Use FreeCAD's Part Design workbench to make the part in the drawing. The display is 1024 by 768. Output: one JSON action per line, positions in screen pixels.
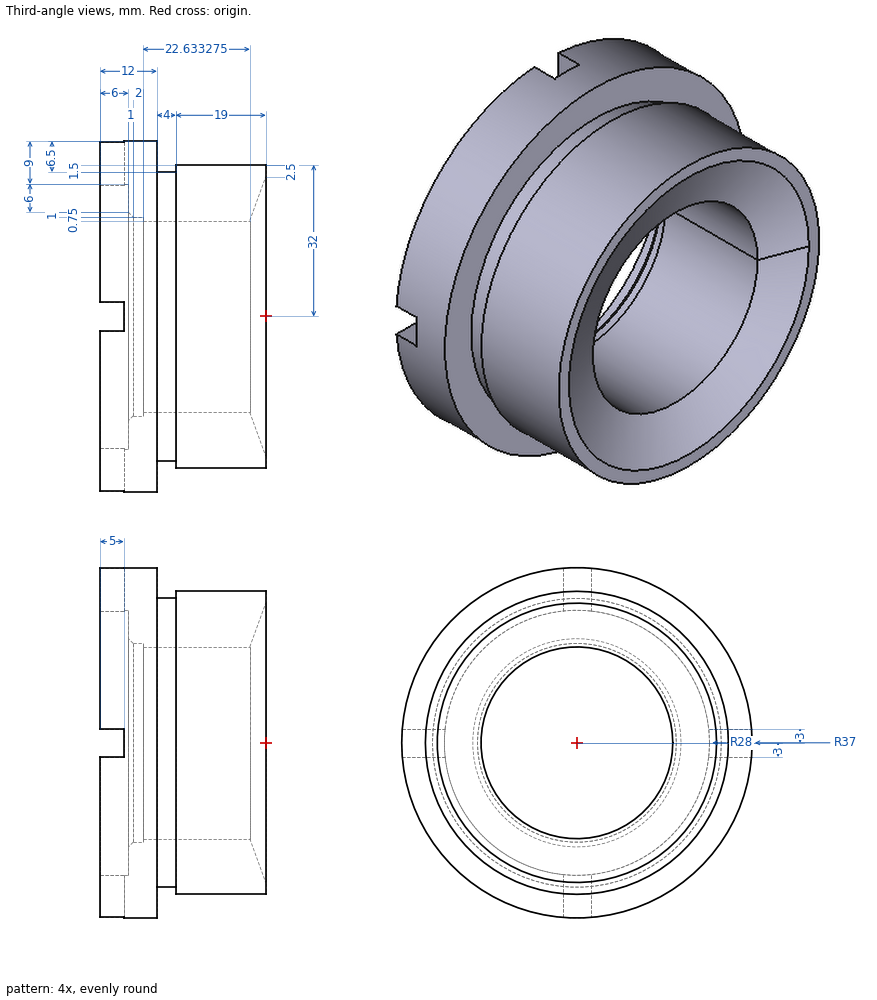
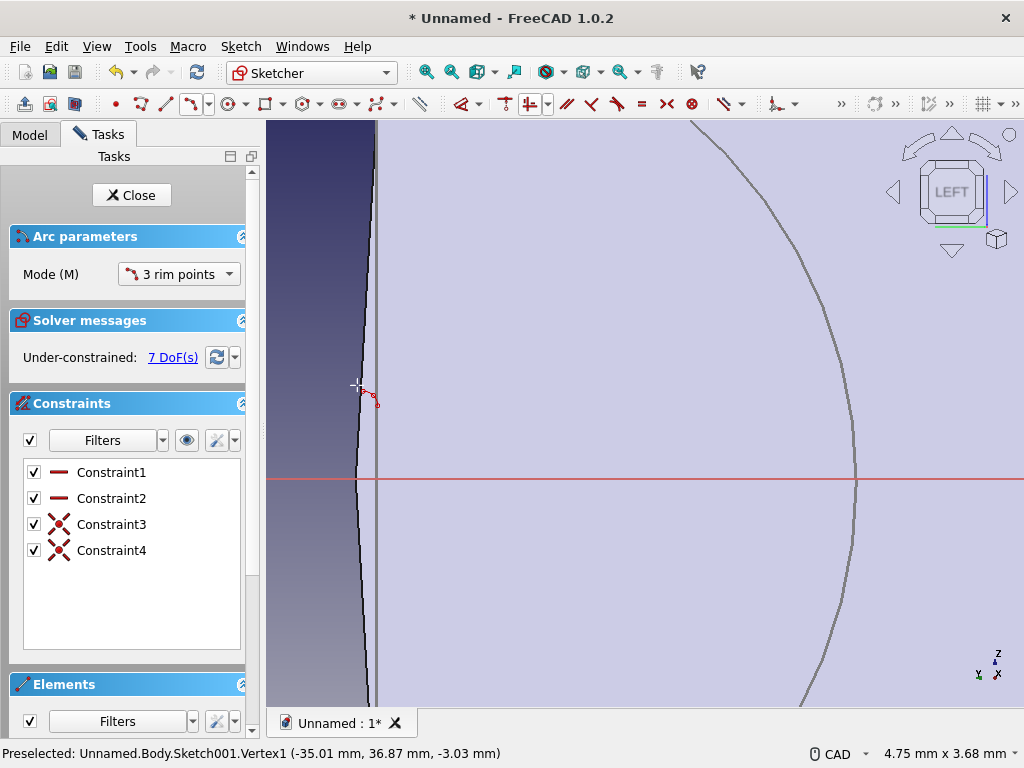
{"action": "left_click", "coordinate": [357, 384]}
{"action": "key", "text": "Escape"}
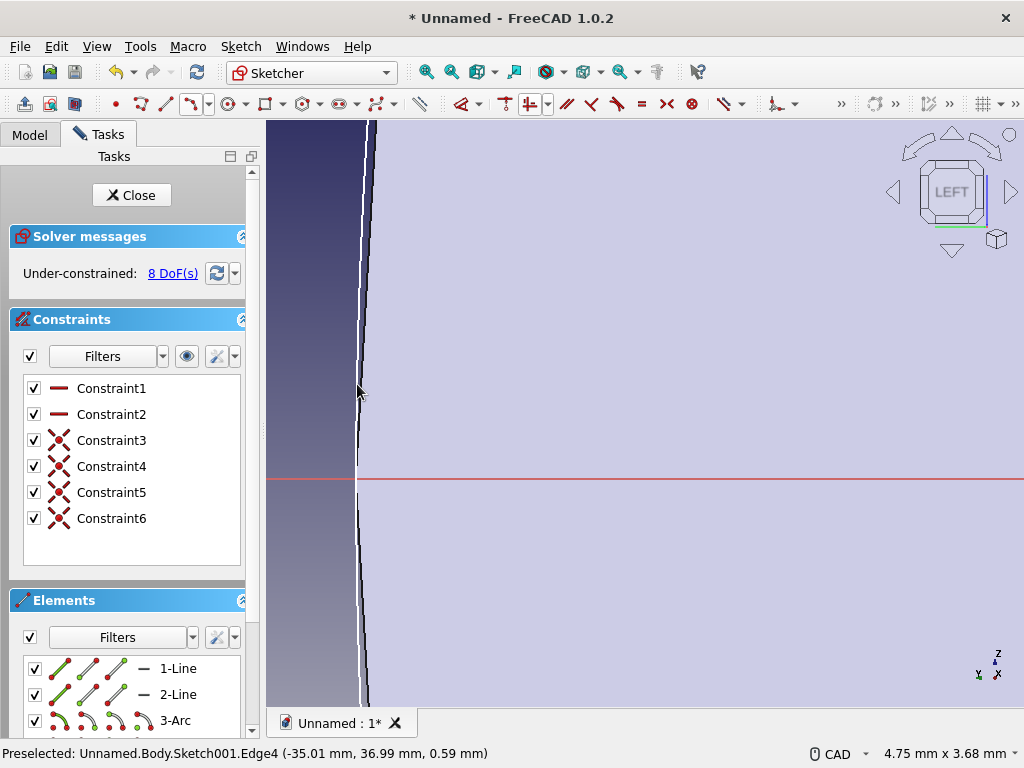
{"action": "scroll", "coordinate": [357, 385], "scroll_direction": "down", "scroll_amount": 6}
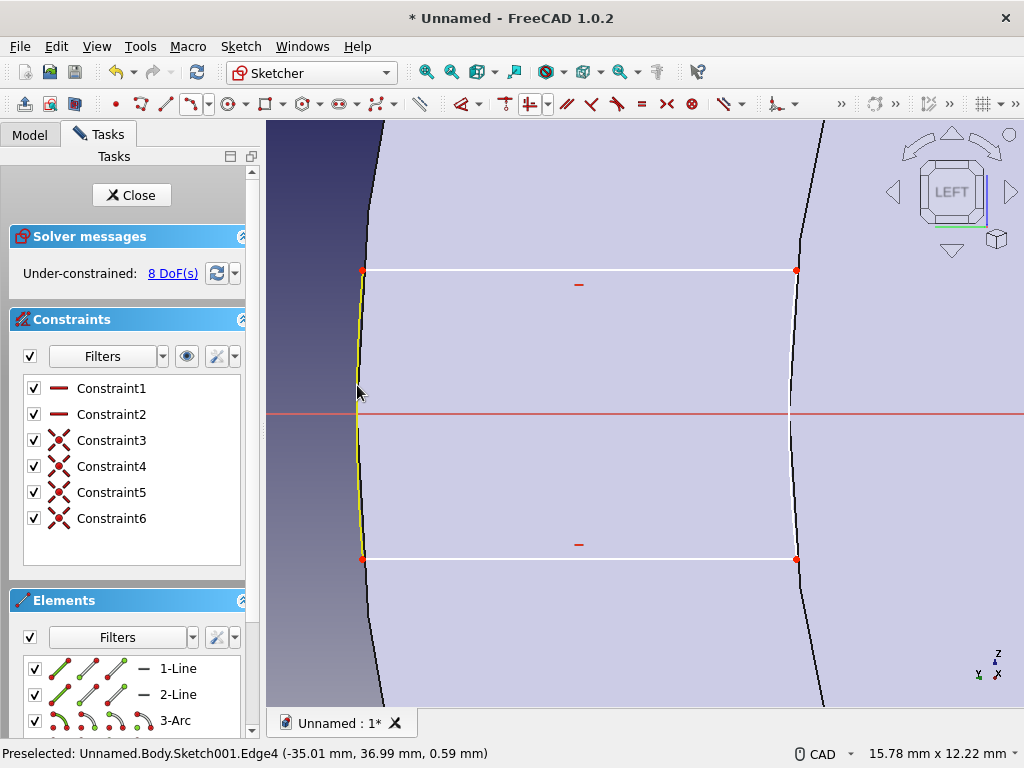
{"action": "left_click", "coordinate": [790, 357]}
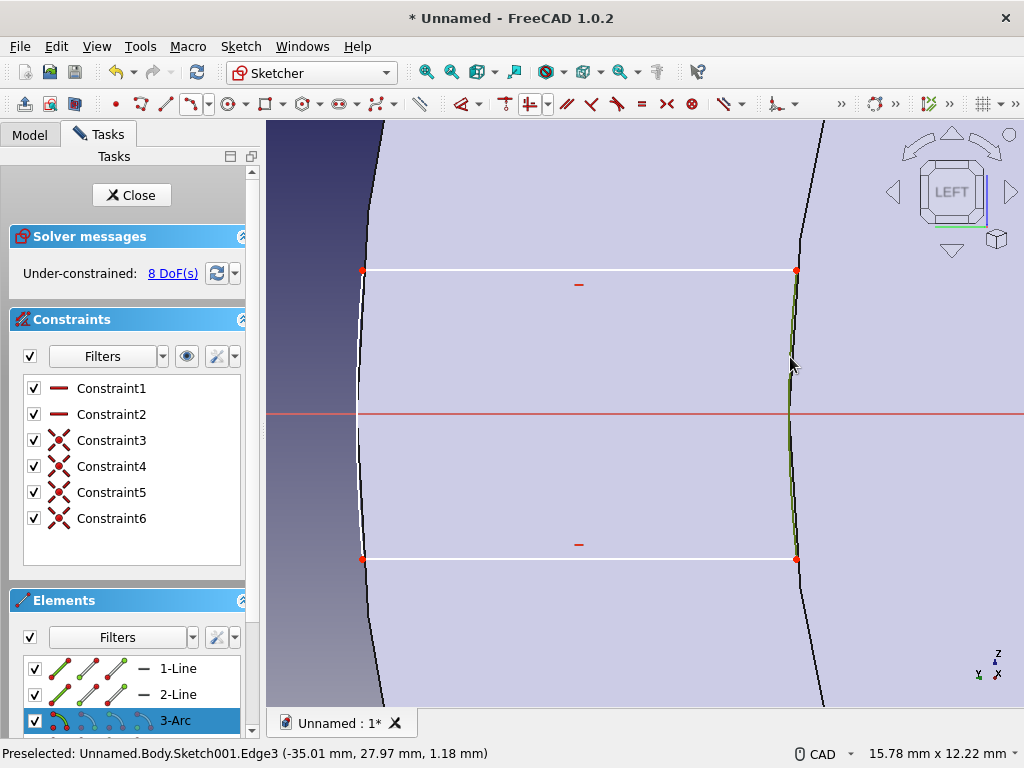
{"action": "left_click", "coordinate": [358, 357]}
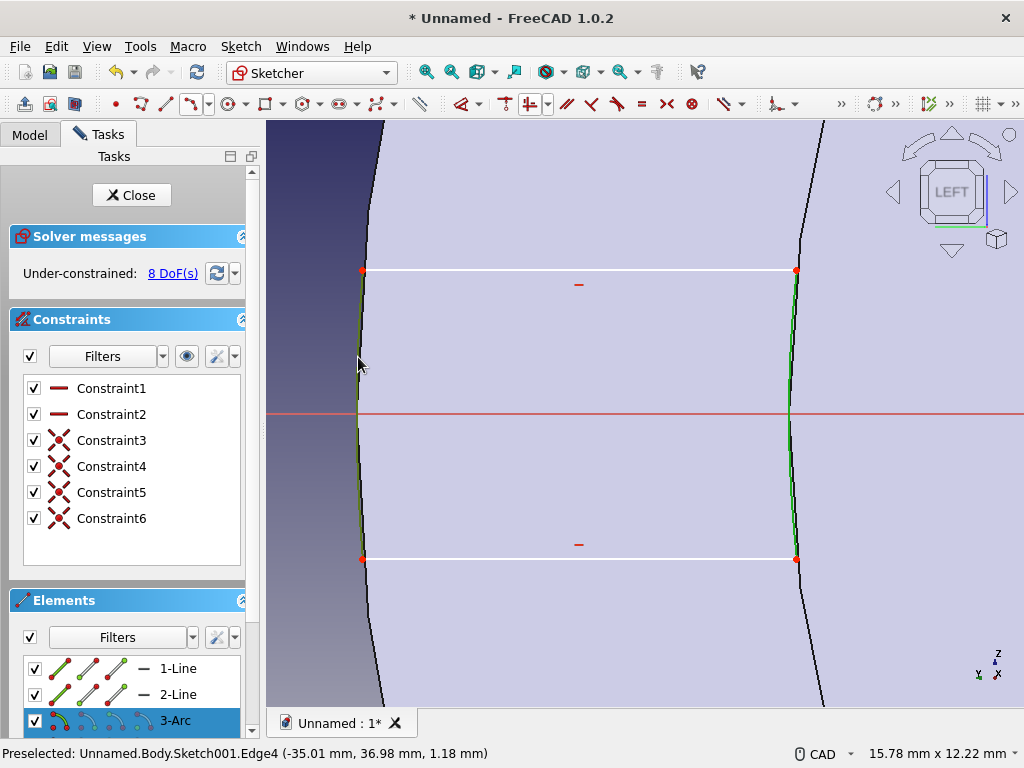
{"action": "left_click", "coordinate": [505, 104]}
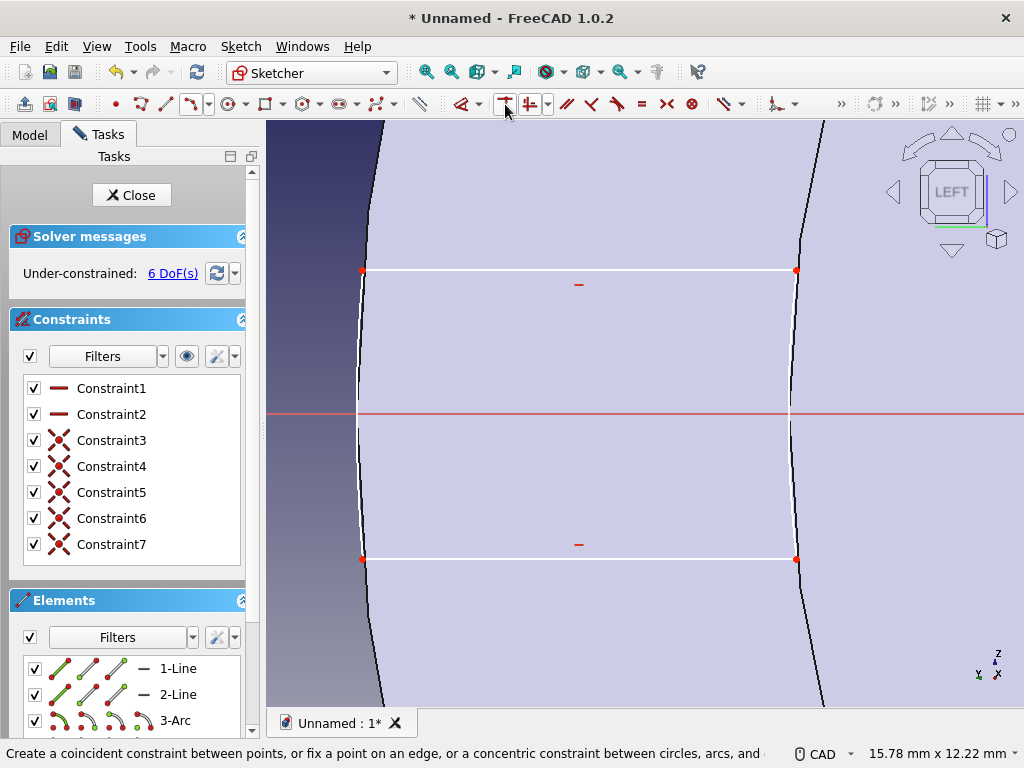
{"action": "scroll", "coordinate": [363, 413], "scroll_direction": "down", "scroll_amount": 7}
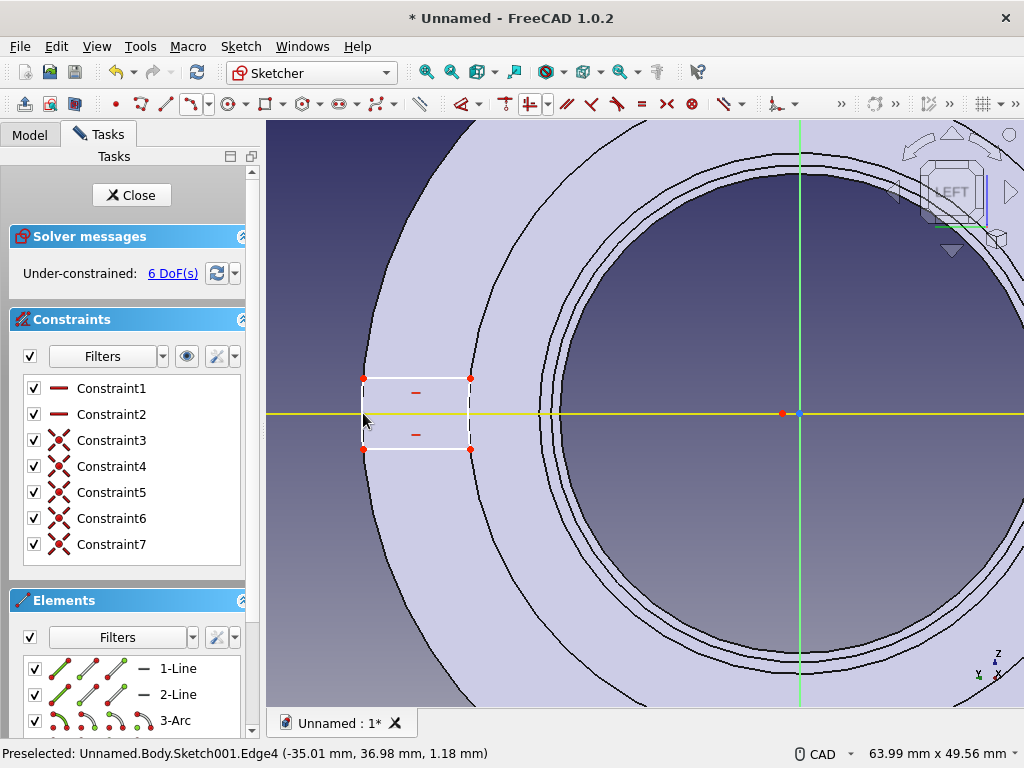
{"action": "left_click_drag", "start_coordinate": [772, 404], "coordinate": [810, 424]}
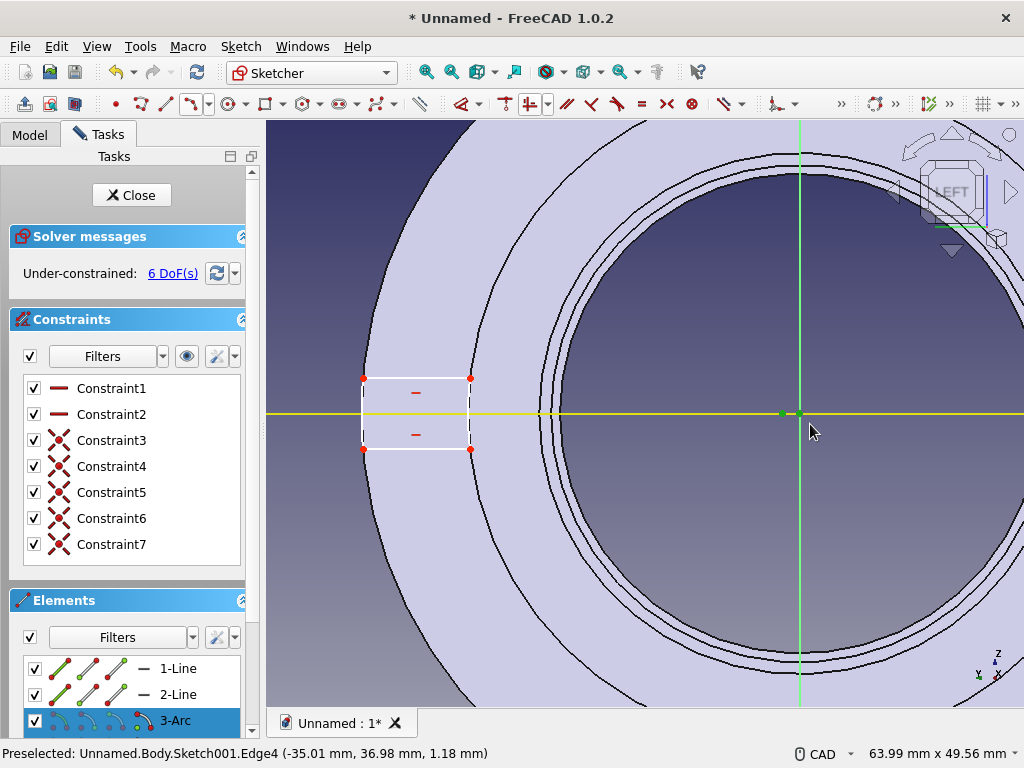
{"action": "left_click", "coordinate": [505, 104]}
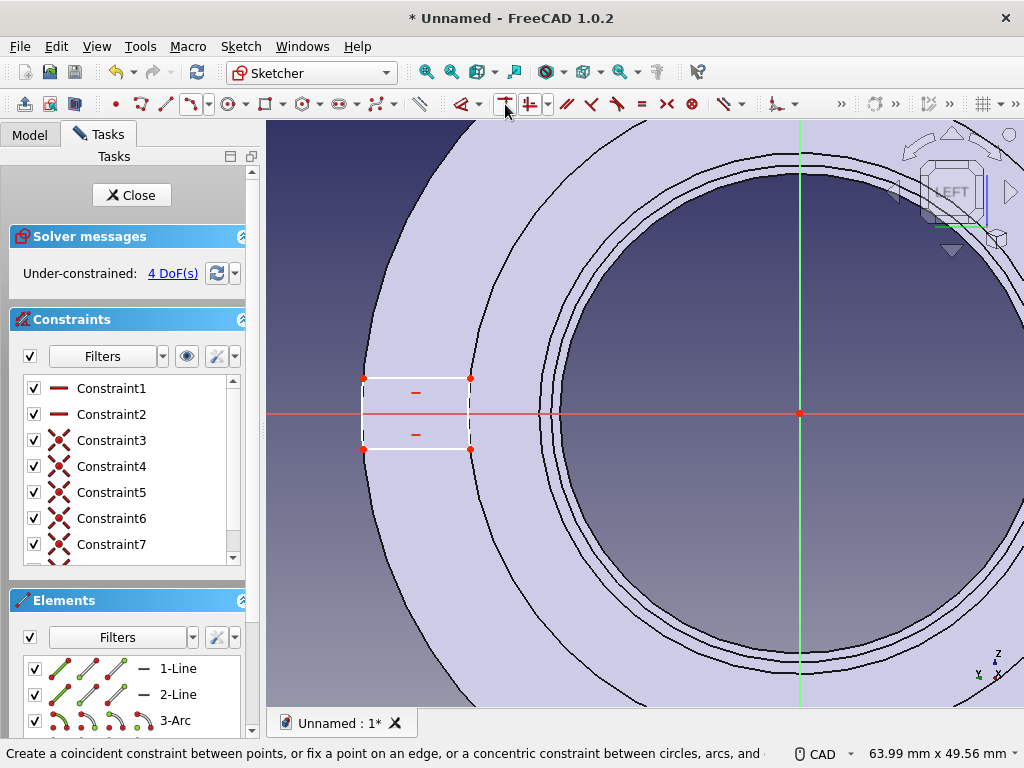
{"action": "left_click", "coordinate": [460, 104]}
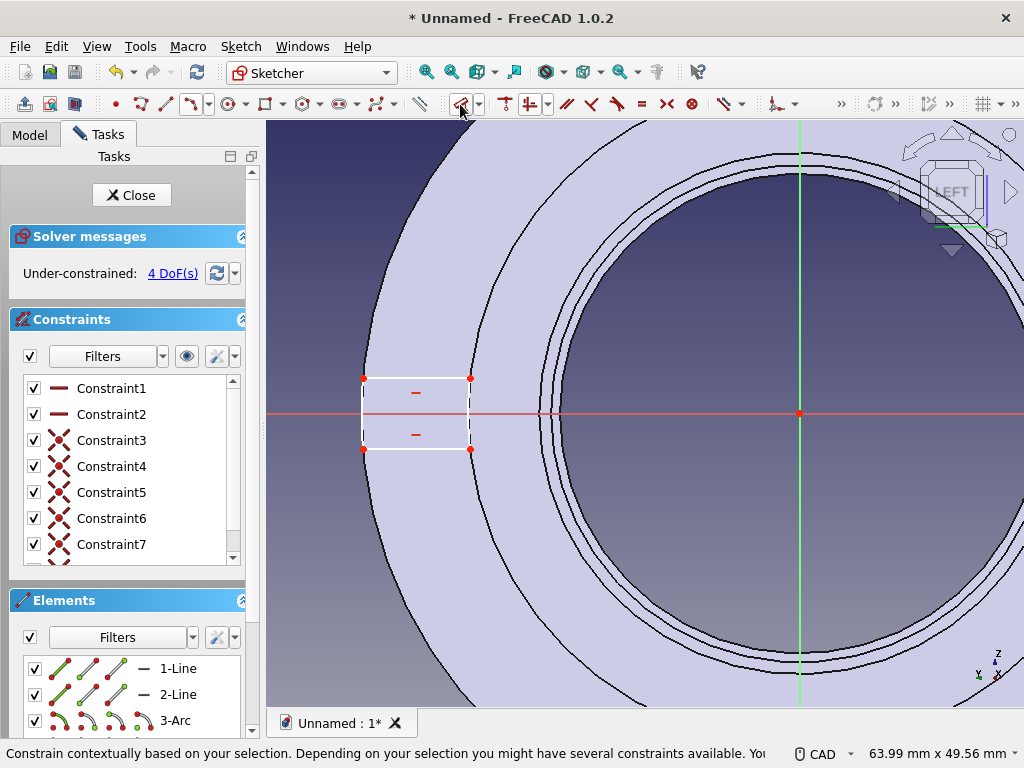
{"action": "left_click", "coordinate": [468, 400]}
{"action": "left_click", "coordinate": [436, 399]}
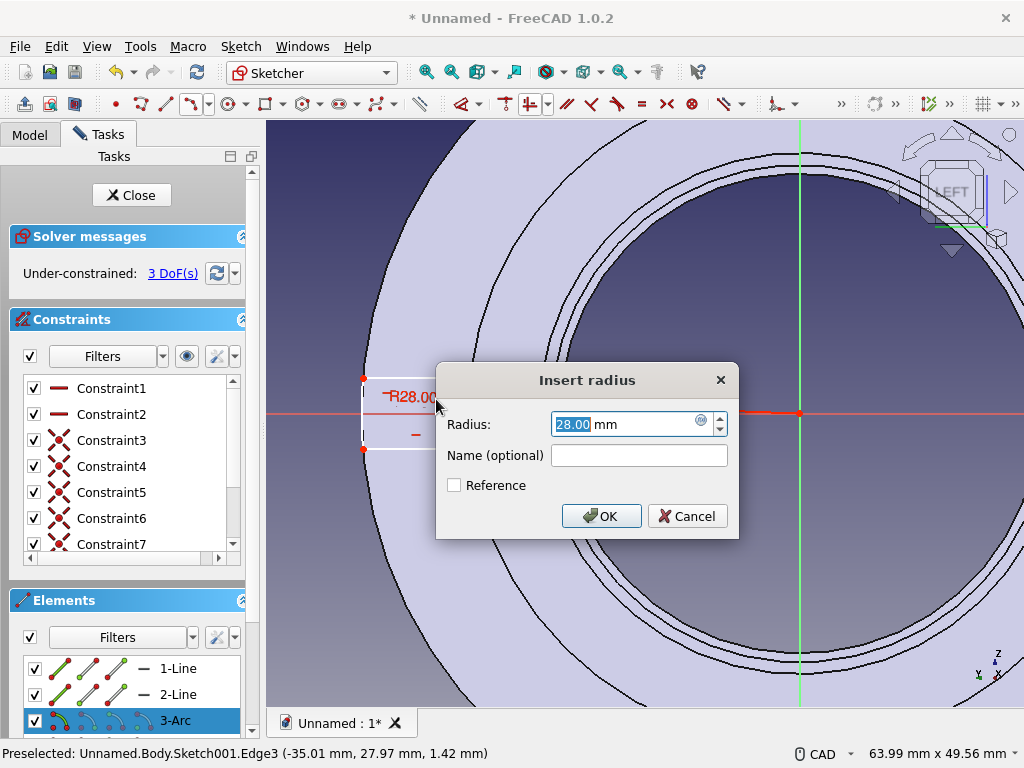
{"action": "type", "text": "28"}
{"action": "key", "text": "Return"}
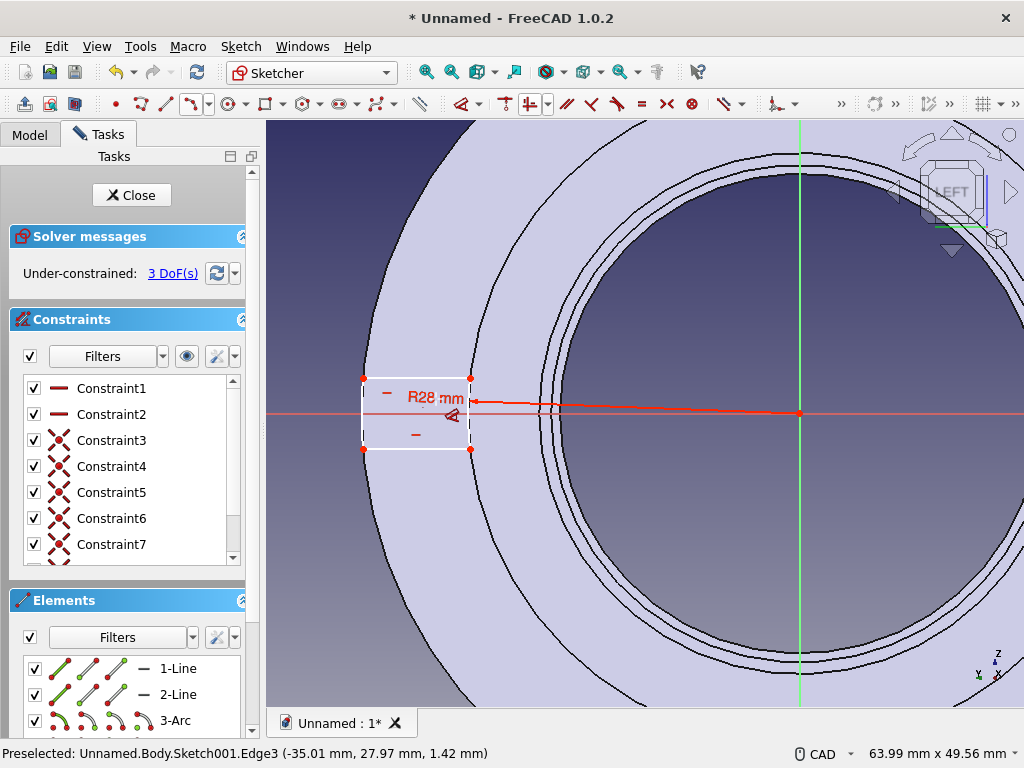
{"action": "left_click", "coordinate": [362, 400]}
{"action": "left_click", "coordinate": [330, 399]}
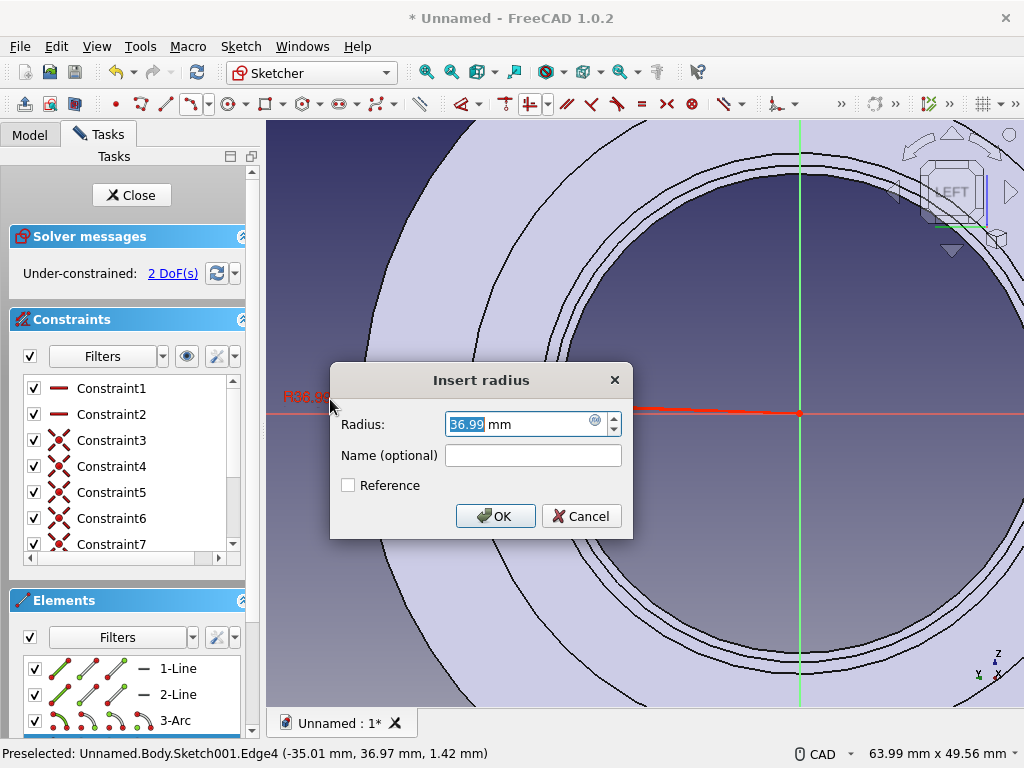
{"action": "type", "text": "37"}
{"action": "key", "text": "Return"}